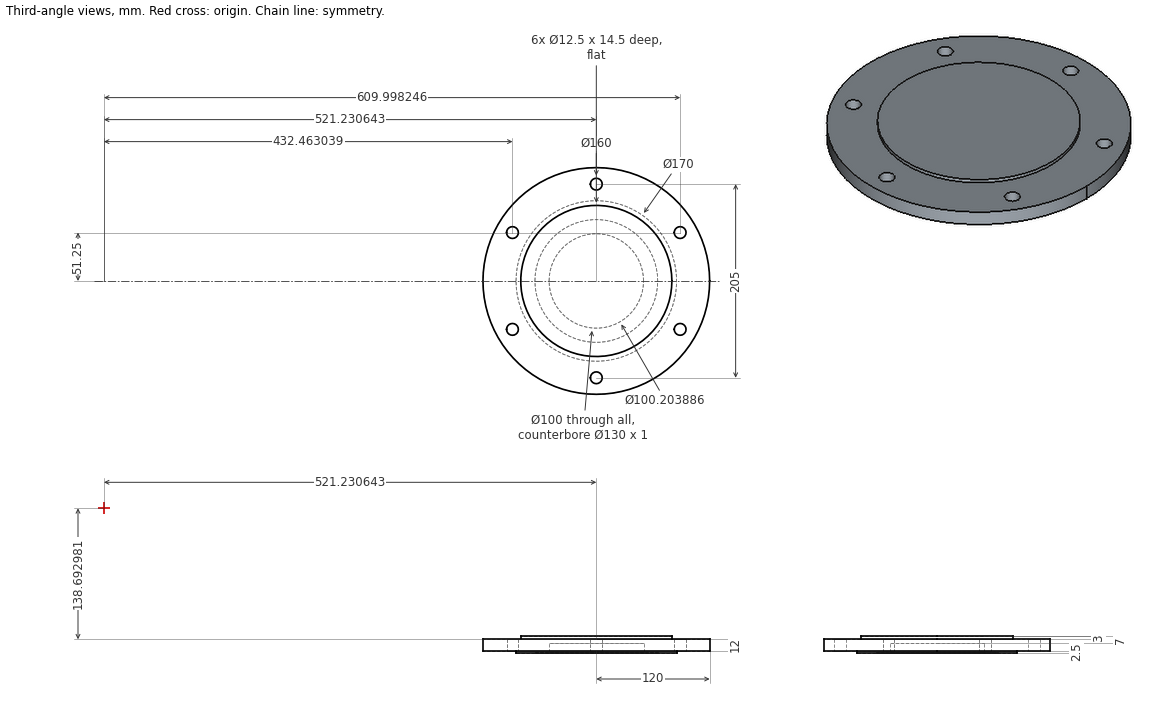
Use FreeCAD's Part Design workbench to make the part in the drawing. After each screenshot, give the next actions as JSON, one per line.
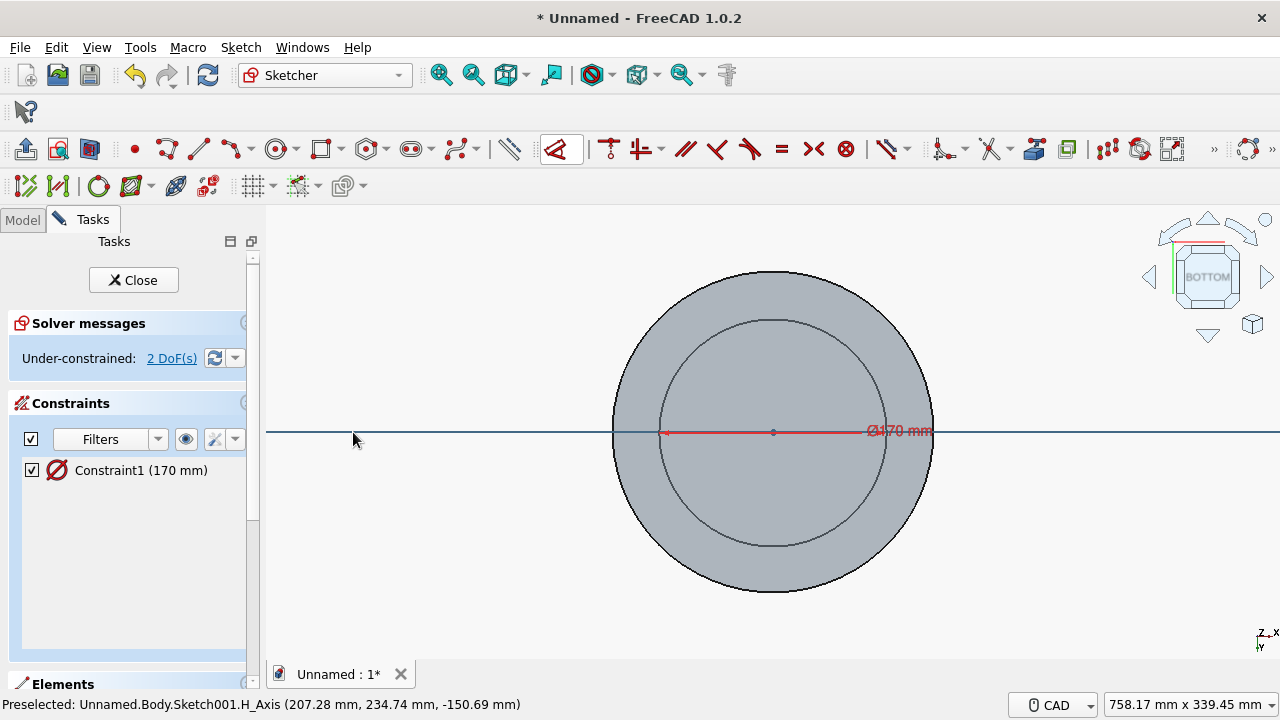
{"action": "key", "text": "c"}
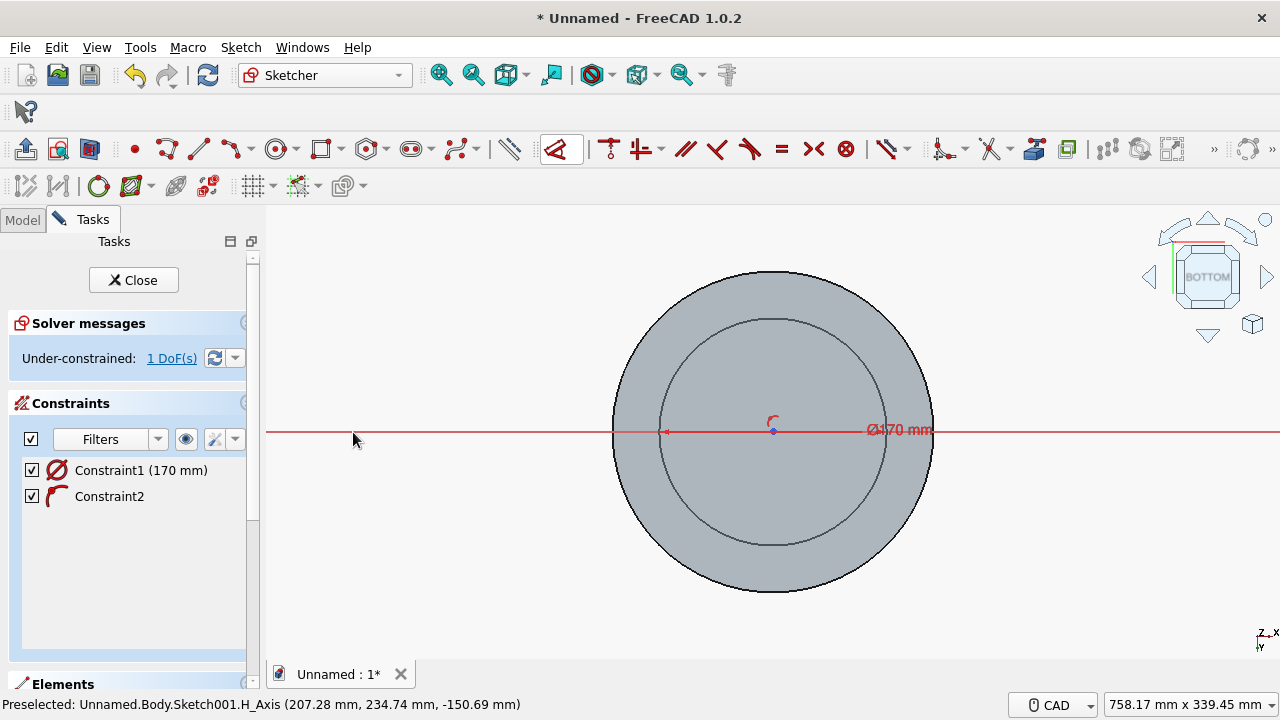
{"action": "key", "text": "d"}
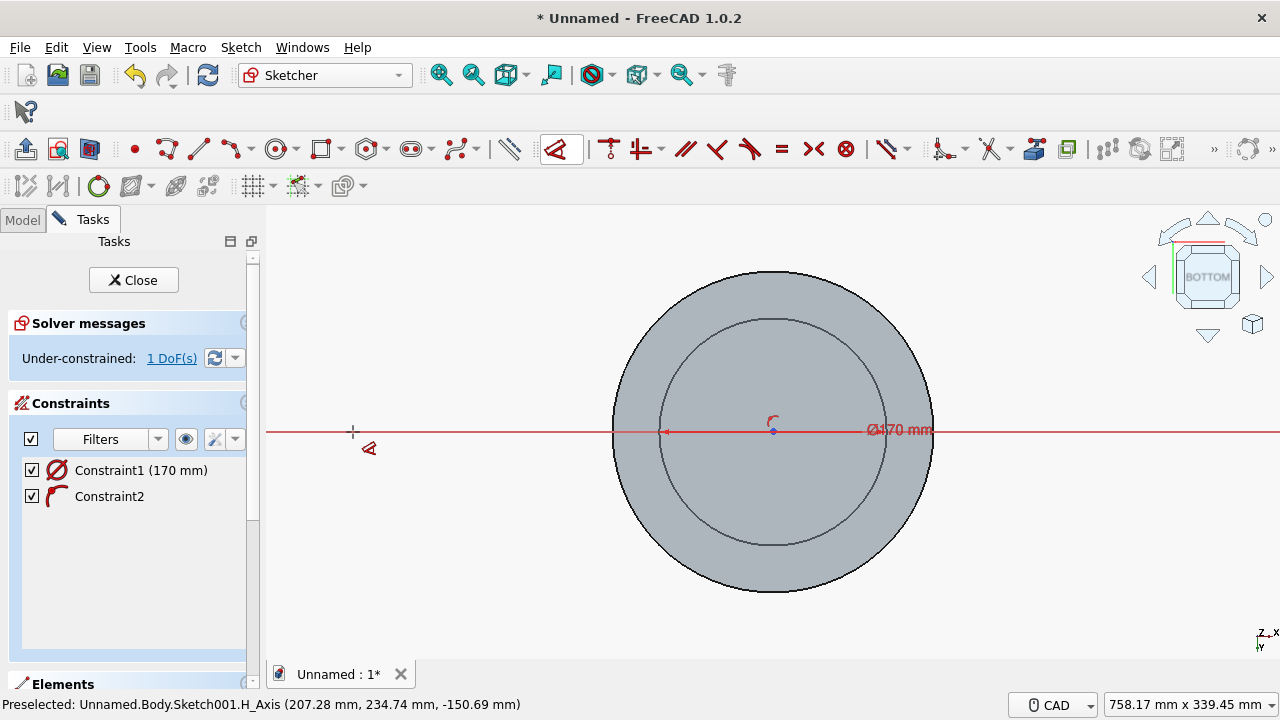
{"action": "left_click", "coordinate": [773, 432]}
{"action": "left_click", "coordinate": [534, 466]}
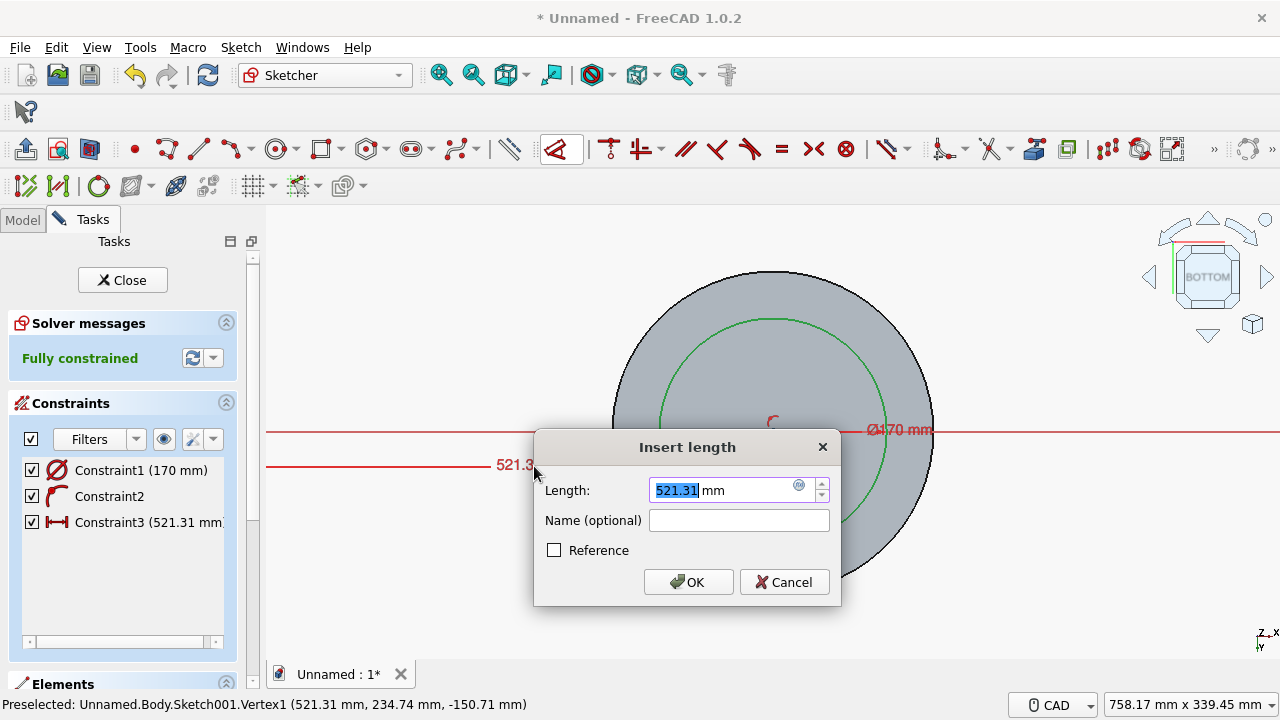
{"action": "type", "text": "521.230643"}
{"action": "key", "text": "Return"}
{"action": "key", "text": "Escape"}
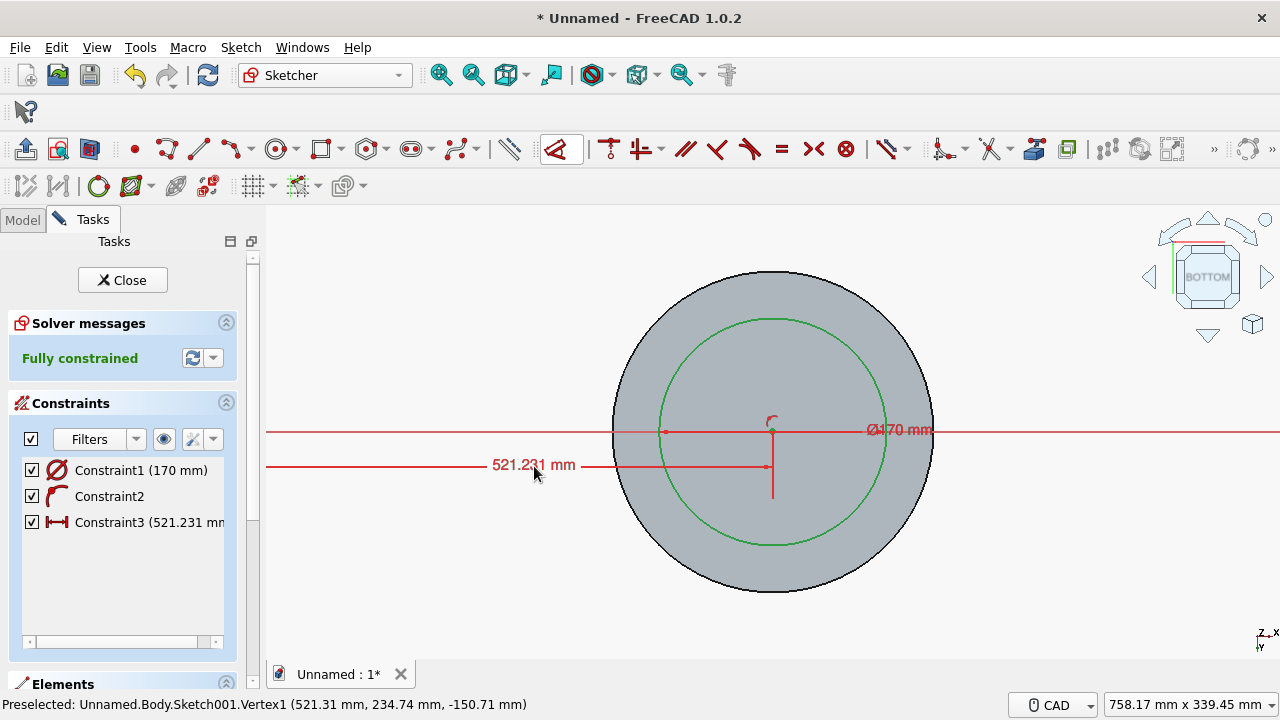
{"action": "left_click", "coordinate": [123, 280]}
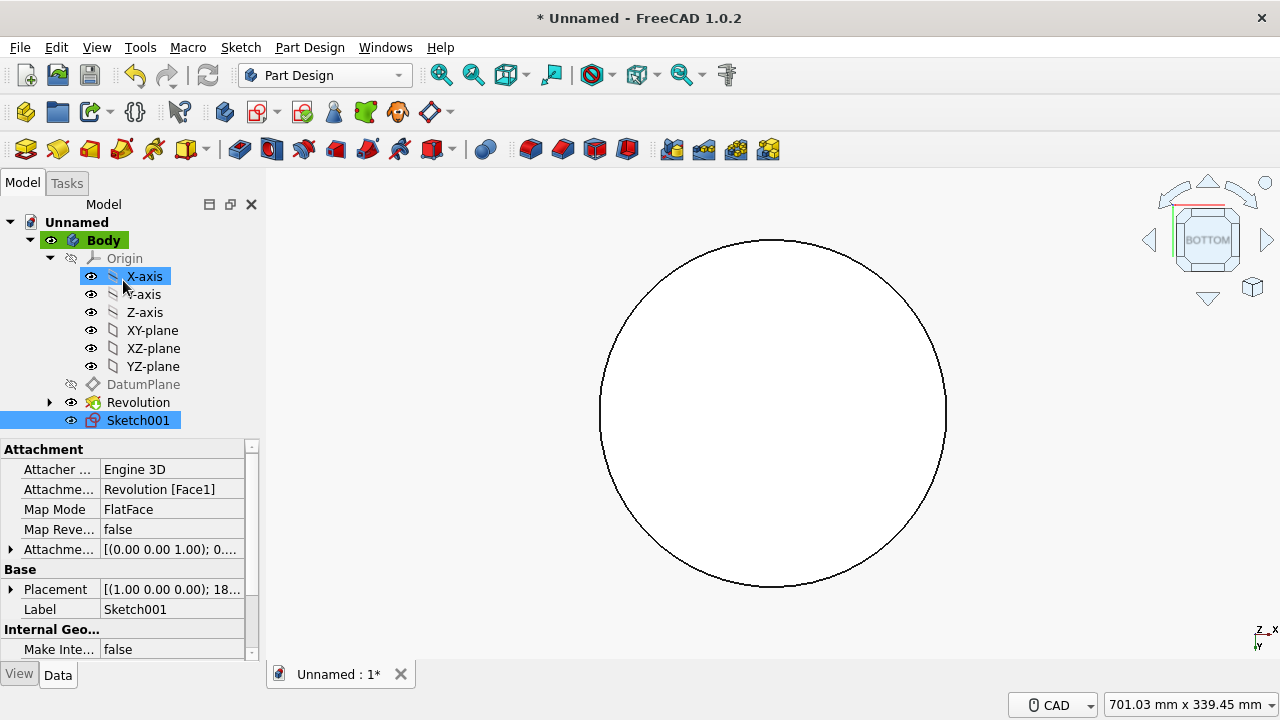
{"action": "left_click", "coordinate": [26, 150]}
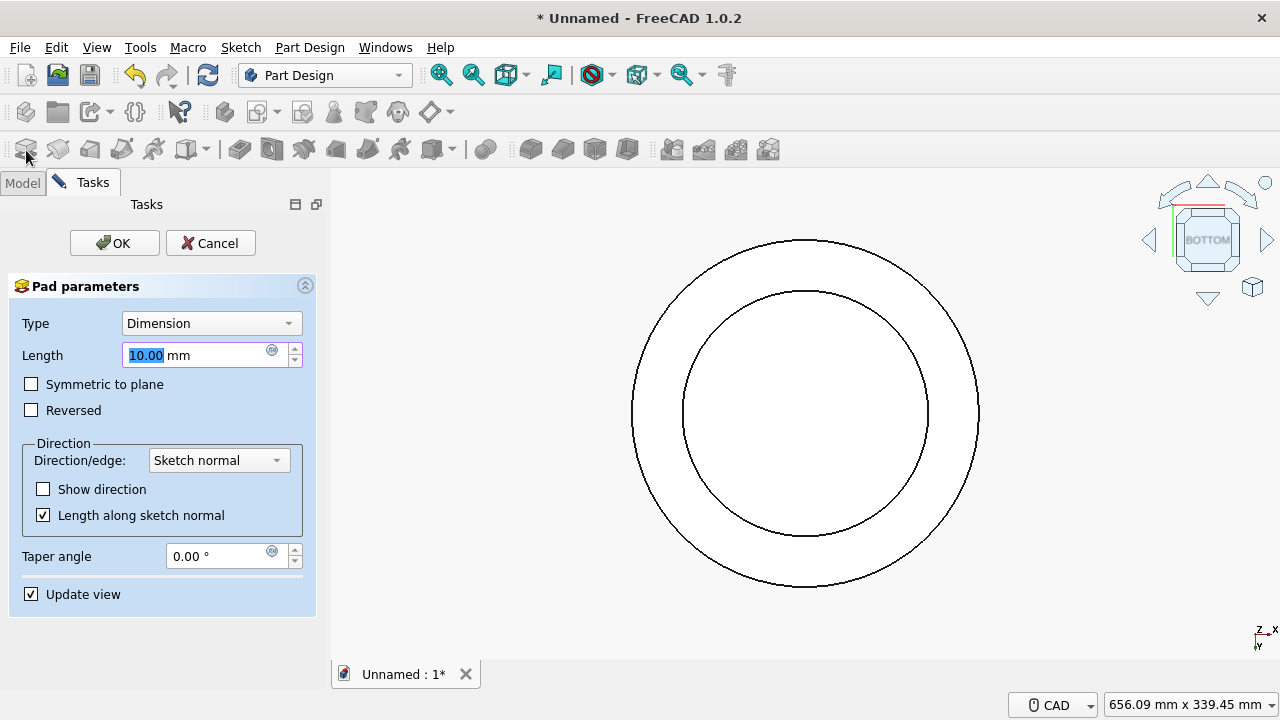
{"action": "type", "text": "2.5"}
{"action": "key", "text": "Tab"}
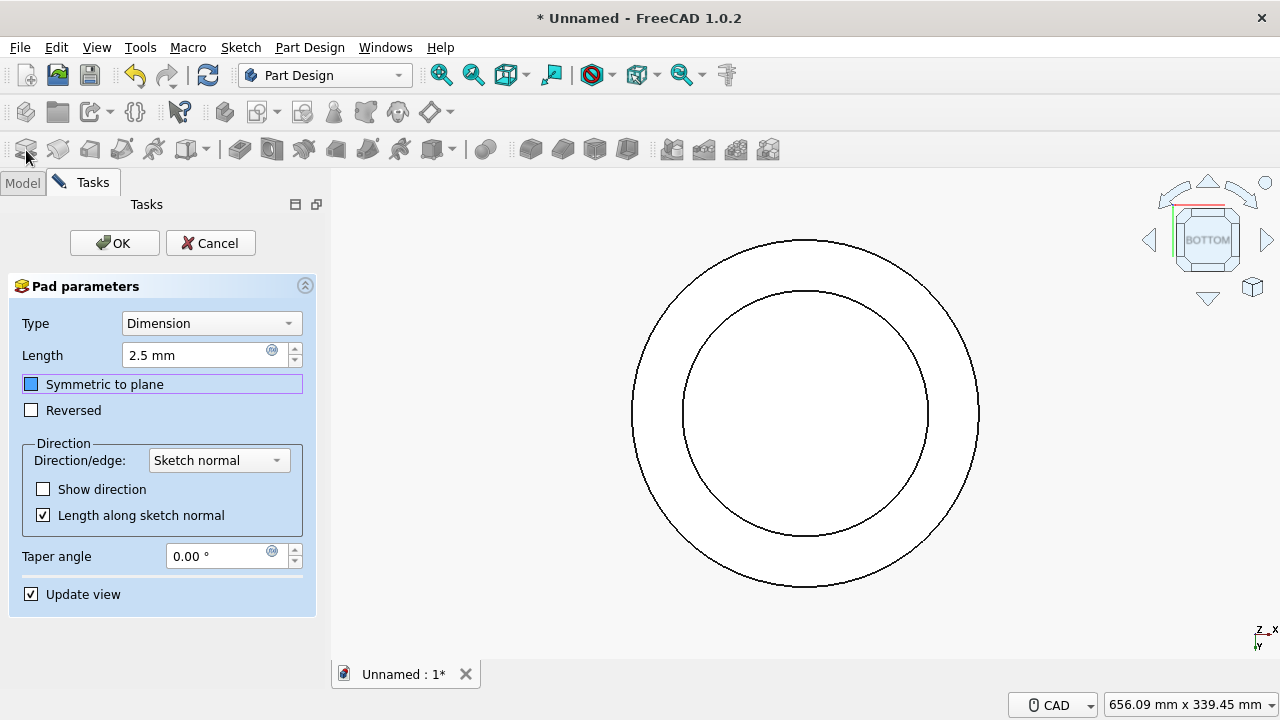
{"action": "left_click", "coordinate": [115, 243]}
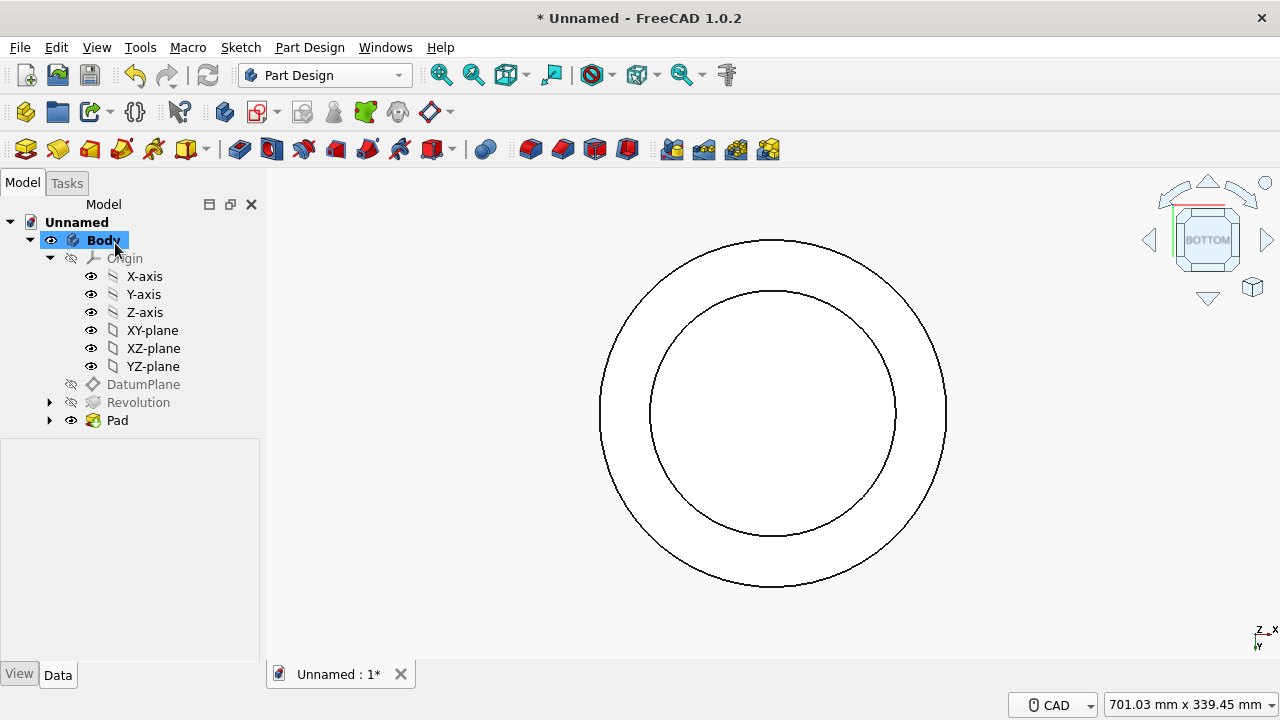
{"action": "key", "text": "0"}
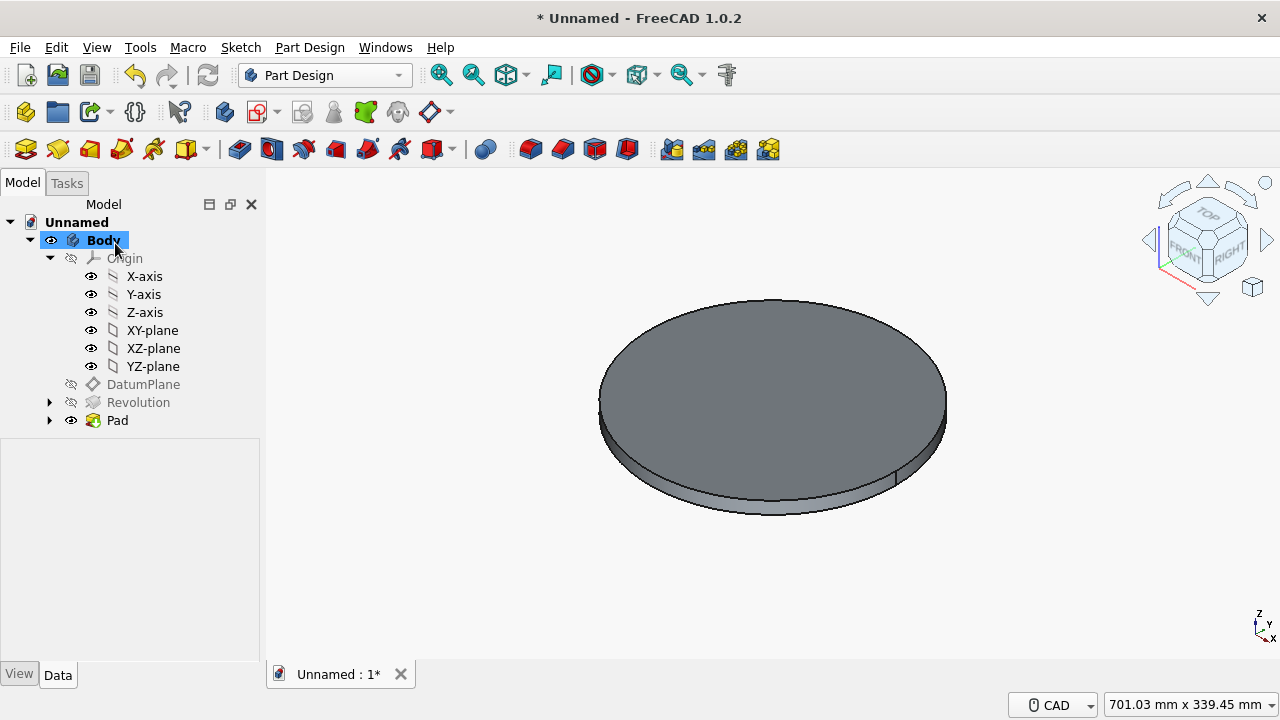
{"action": "left_click", "coordinate": [773, 399]}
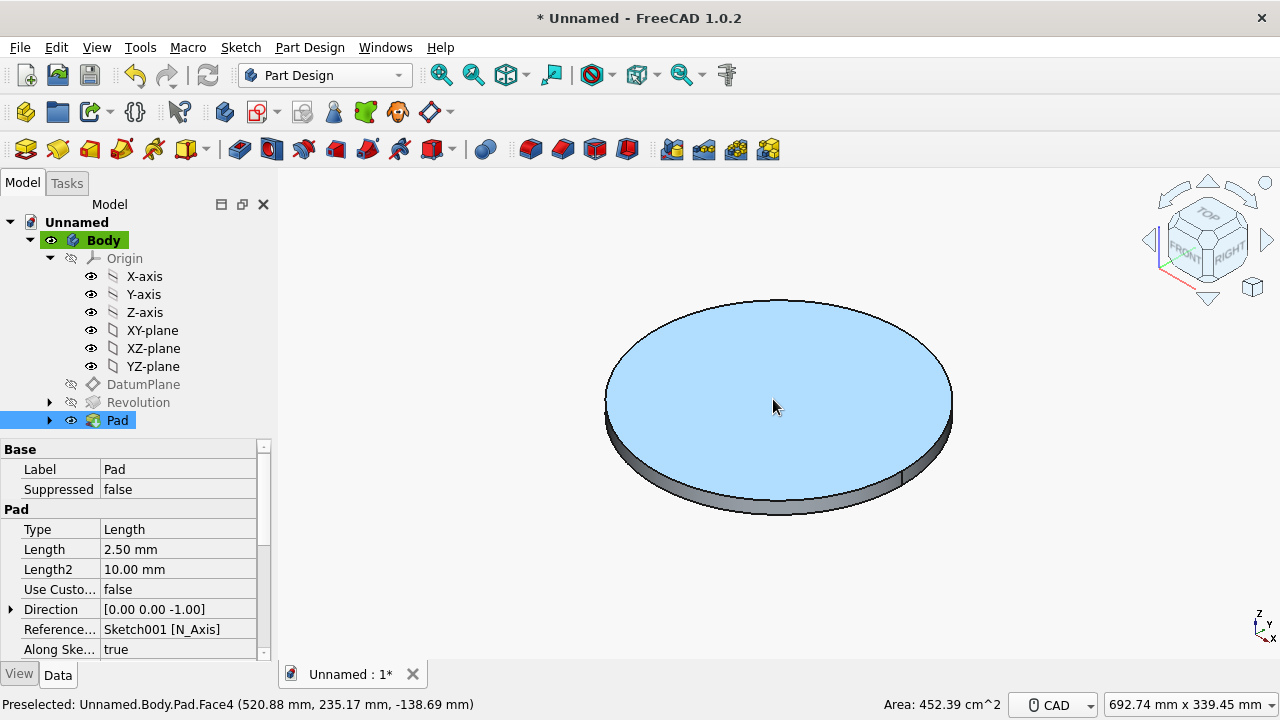
{"action": "left_click", "coordinate": [258, 112]}